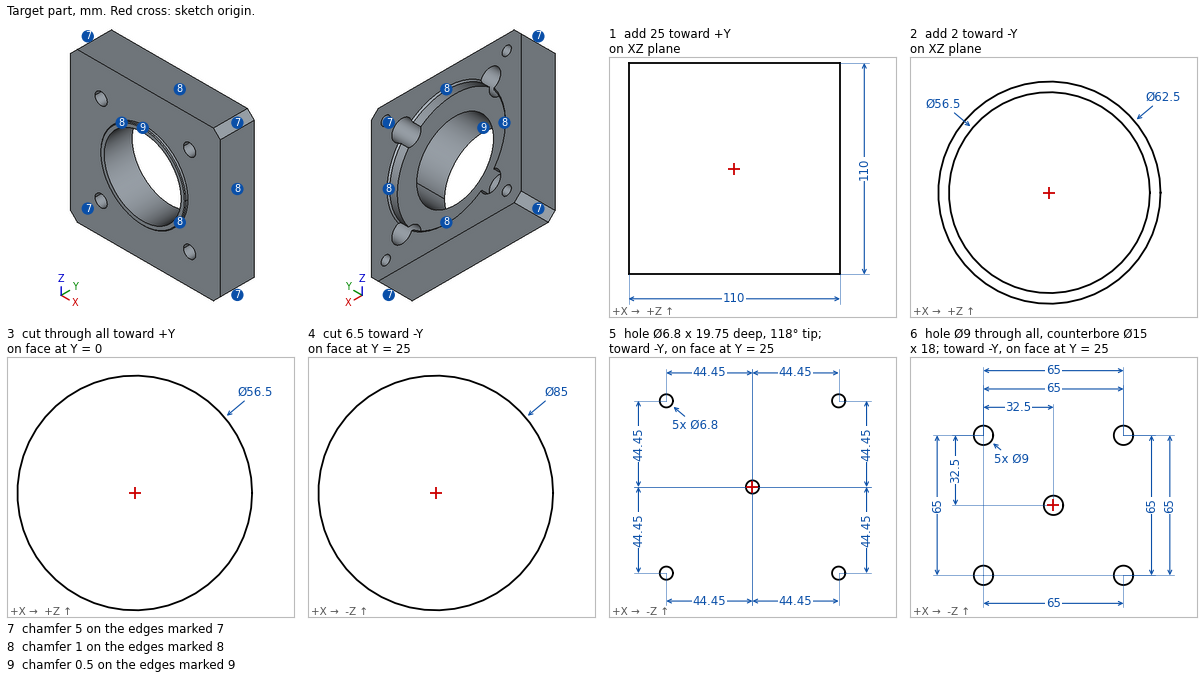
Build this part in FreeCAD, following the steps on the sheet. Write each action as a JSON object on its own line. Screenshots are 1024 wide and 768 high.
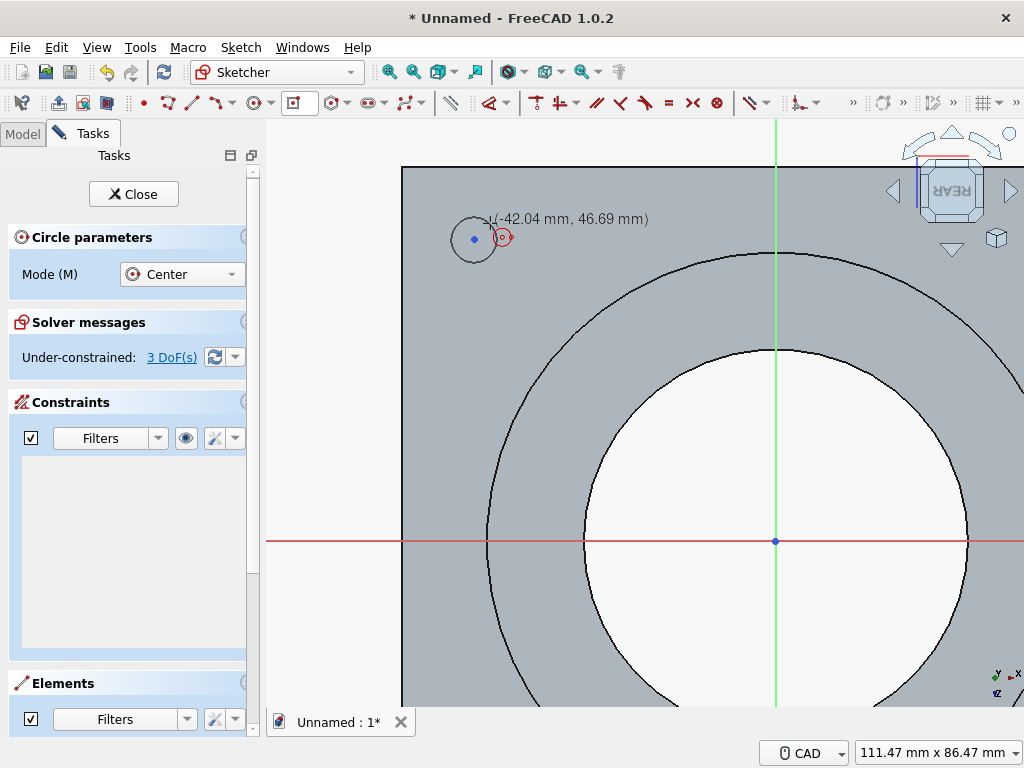
{"action": "left_click", "coordinate": [776, 541]}
{"action": "left_click", "coordinate": [792, 525]}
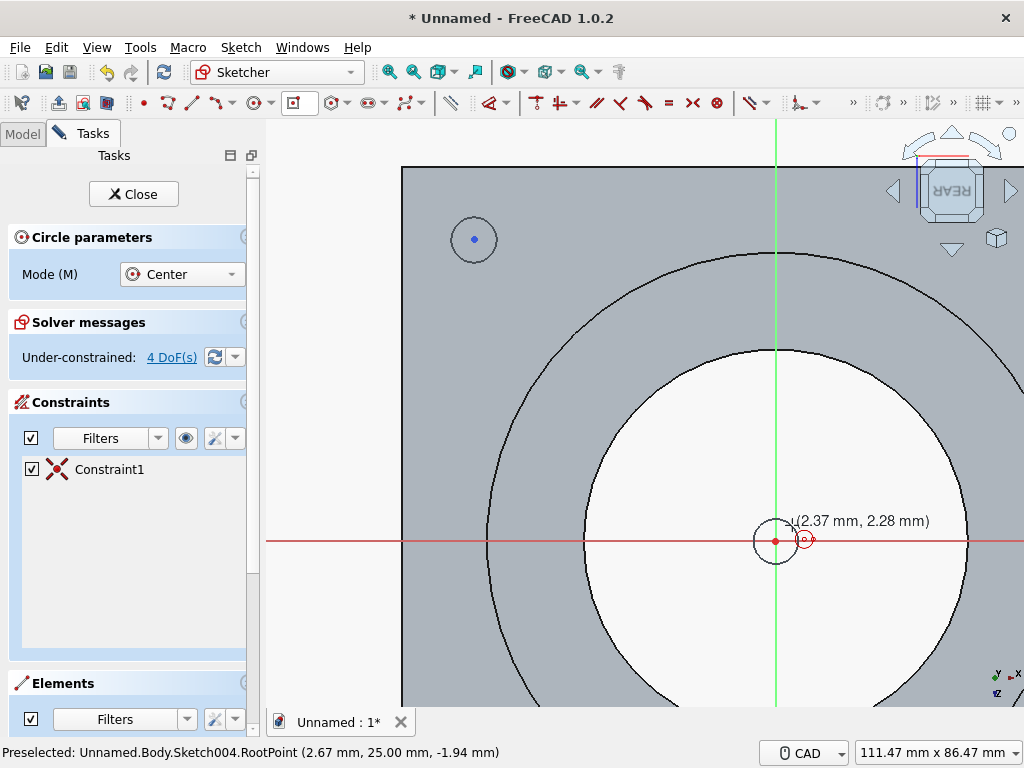
{"action": "scroll", "coordinate": [334, 257], "scroll_direction": "down", "scroll_amount": 3}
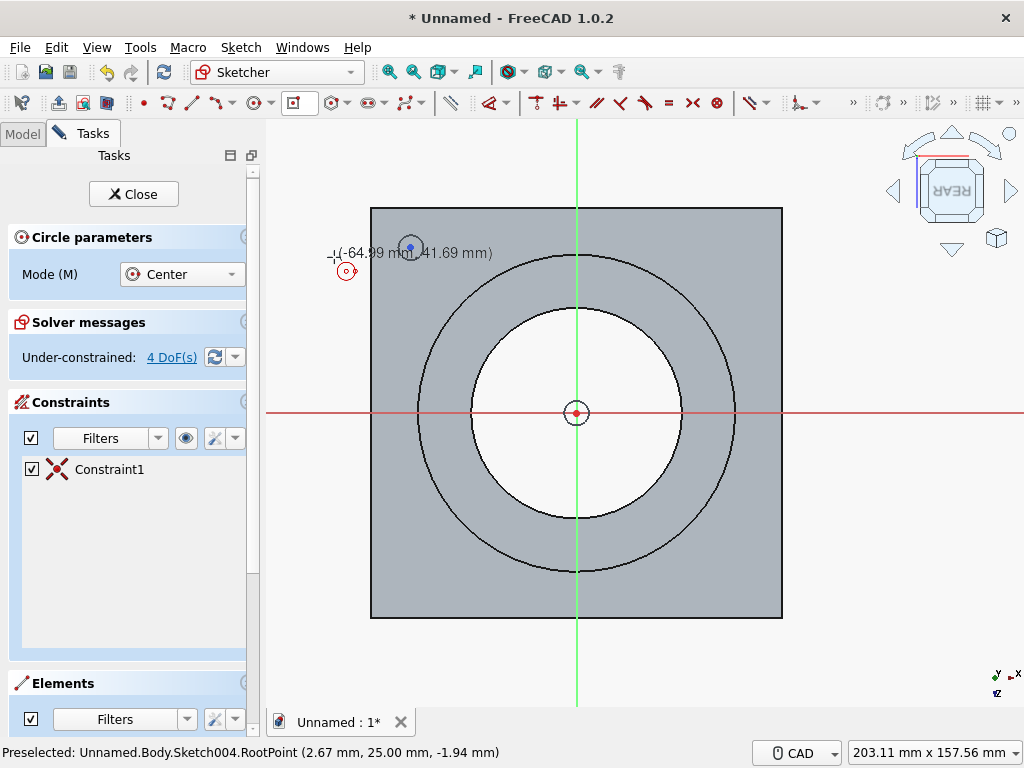
{"action": "scroll", "coordinate": [742, 247], "scroll_direction": "up", "scroll_amount": 3}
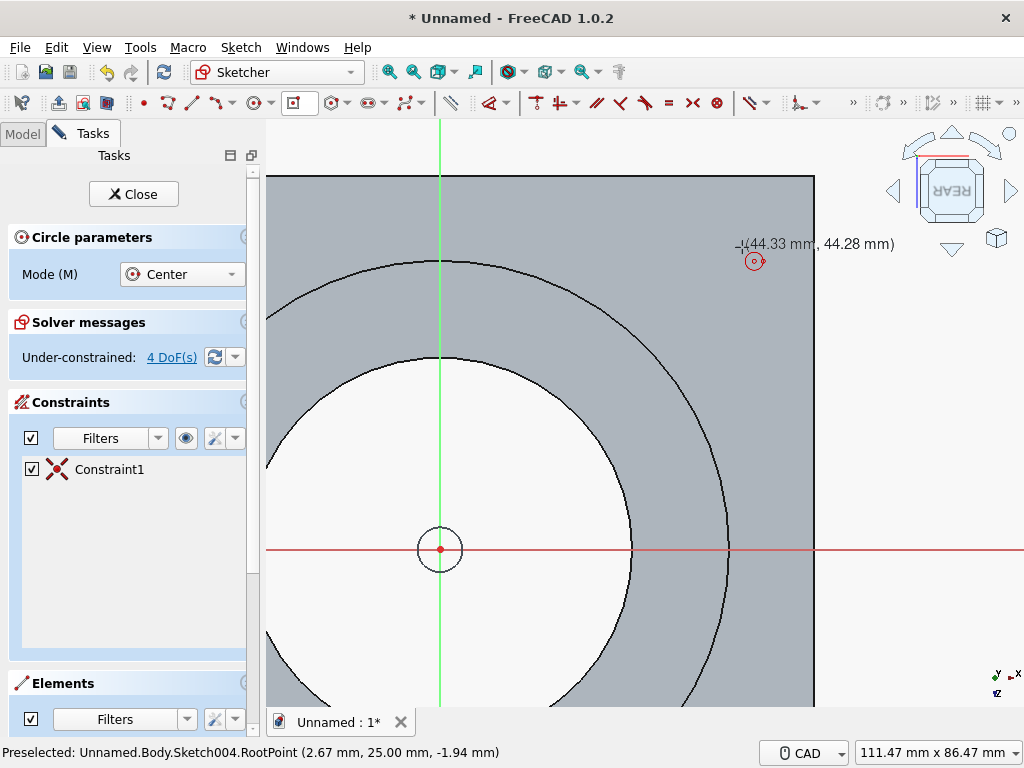
{"action": "left_click", "coordinate": [742, 247]}
{"action": "left_click", "coordinate": [759, 231]}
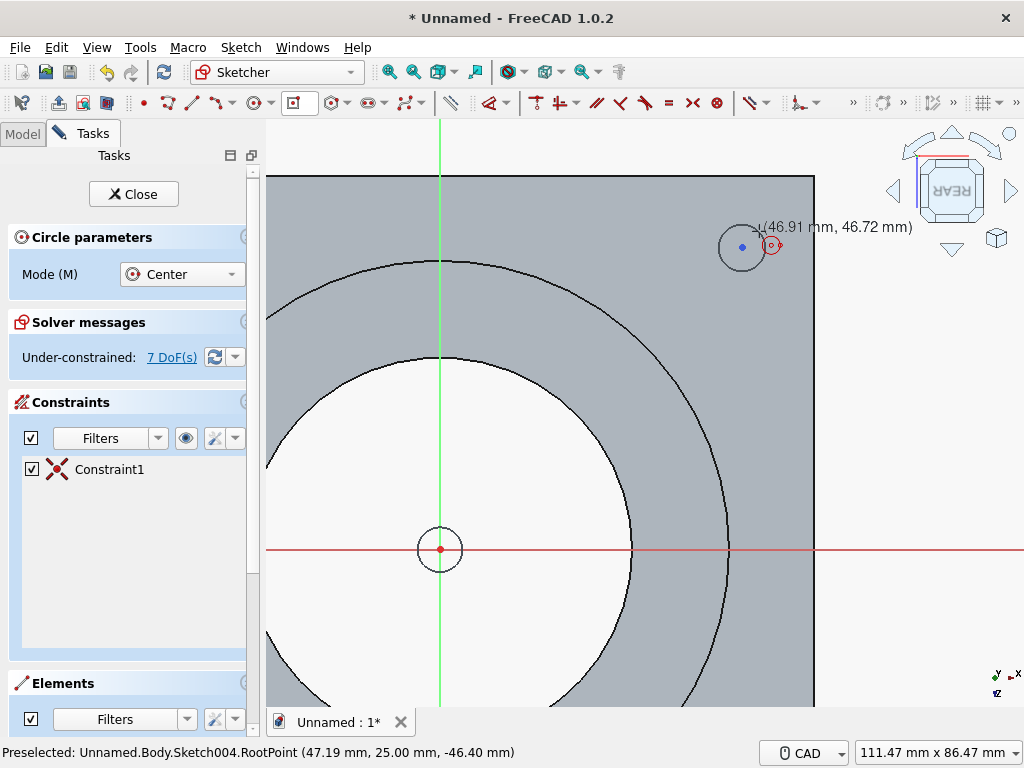
{"action": "scroll", "coordinate": [742, 247], "scroll_direction": "down", "scroll_amount": 3}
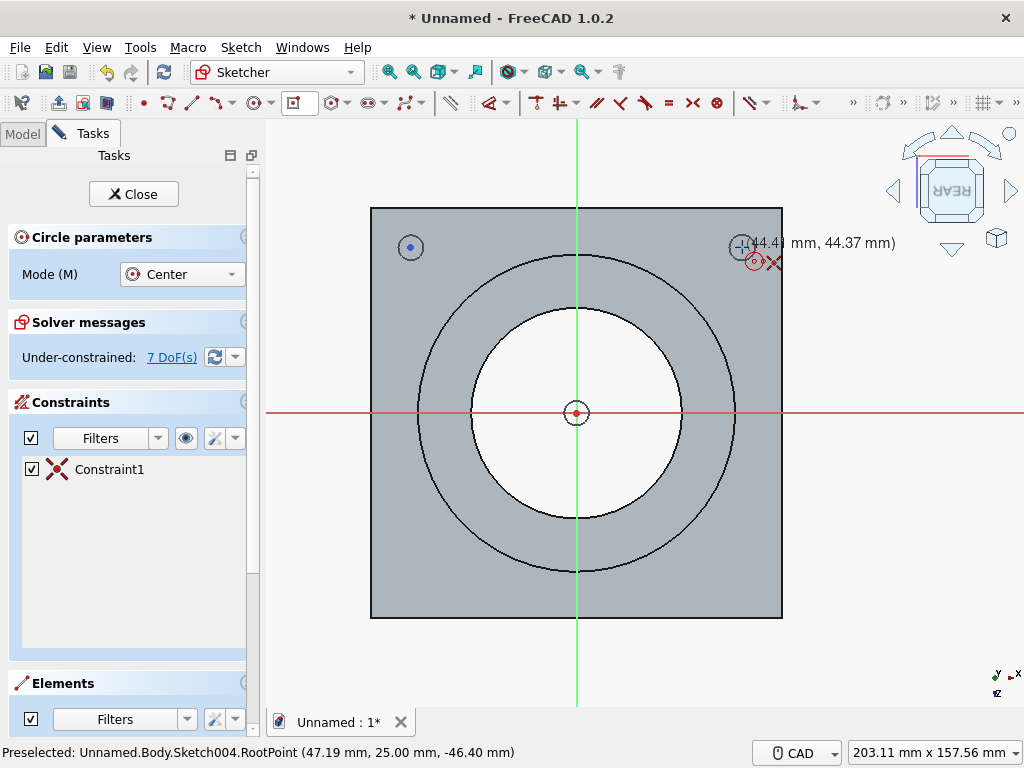
{"action": "scroll", "coordinate": [411, 579], "scroll_direction": "up", "scroll_amount": 3}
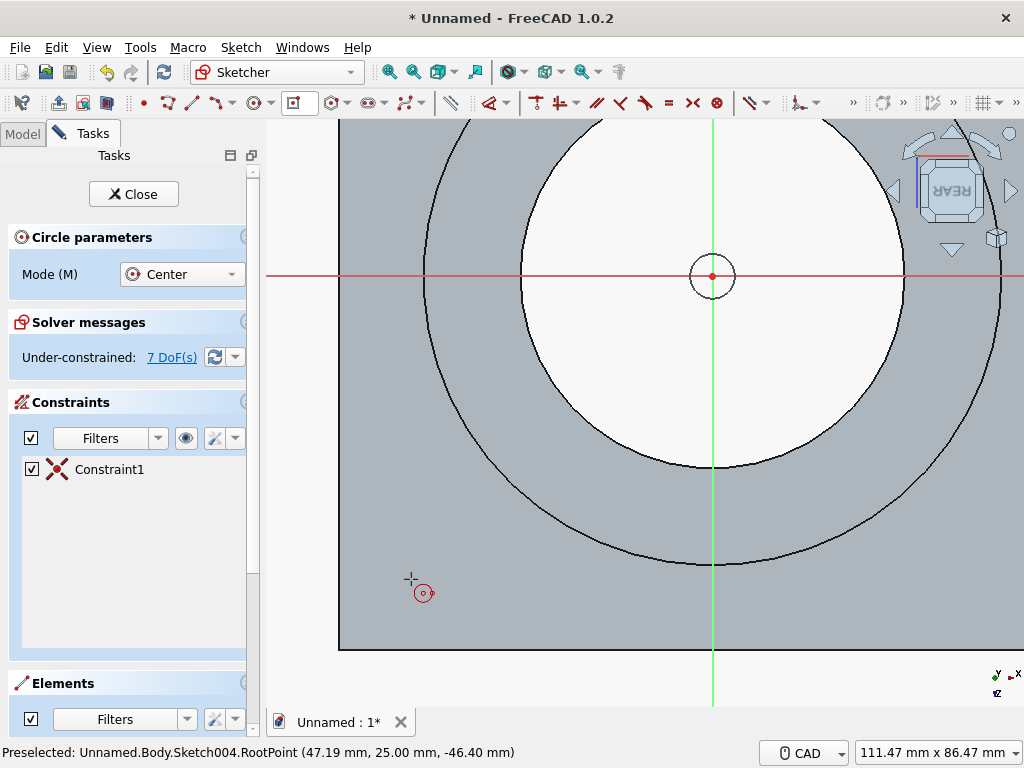
{"action": "left_click", "coordinate": [410, 579]}
{"action": "left_click", "coordinate": [427, 562]}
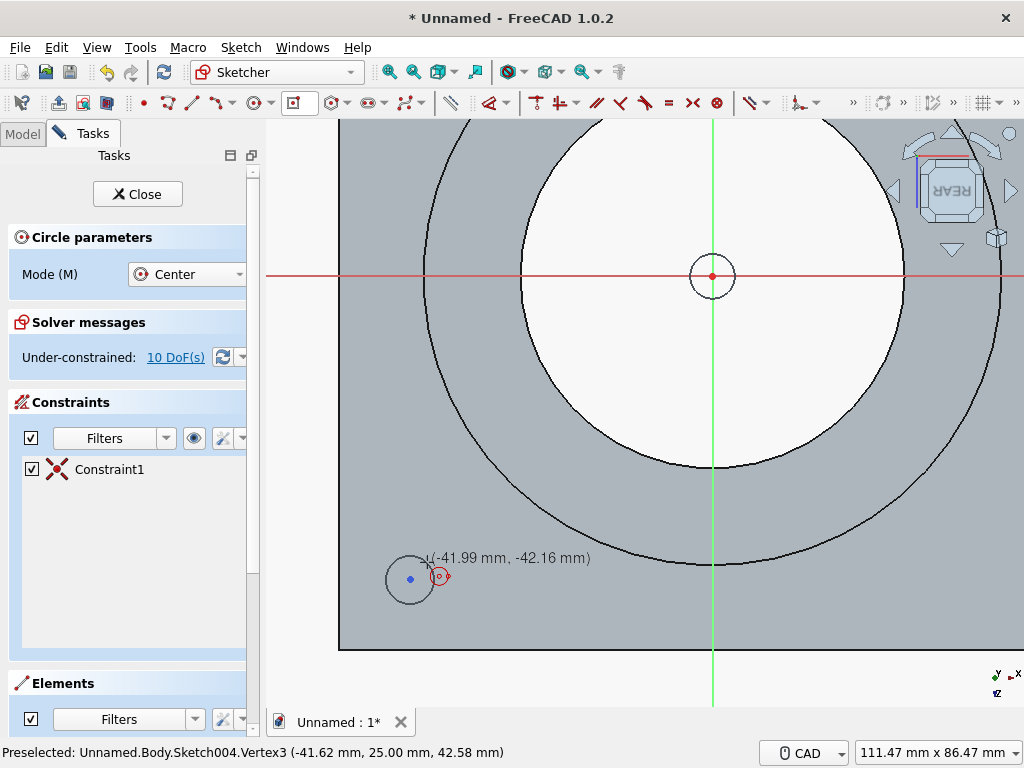
{"action": "scroll", "coordinate": [411, 579], "scroll_direction": "down", "scroll_amount": 3}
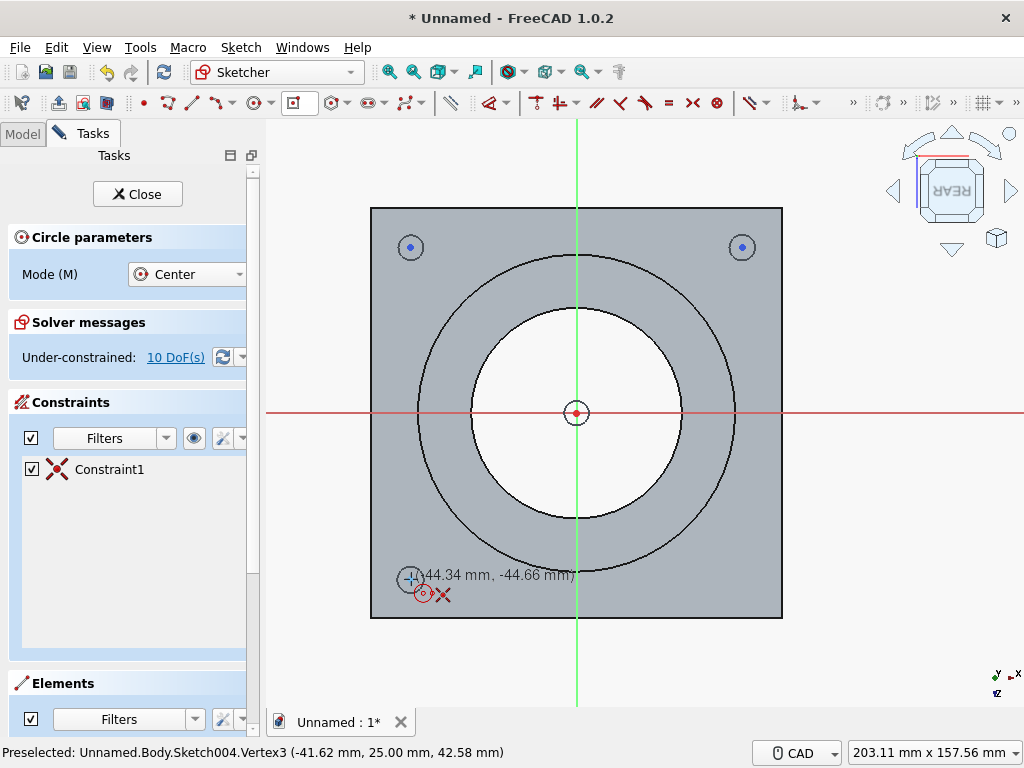
{"action": "scroll", "coordinate": [742, 579], "scroll_direction": "up", "scroll_amount": 3}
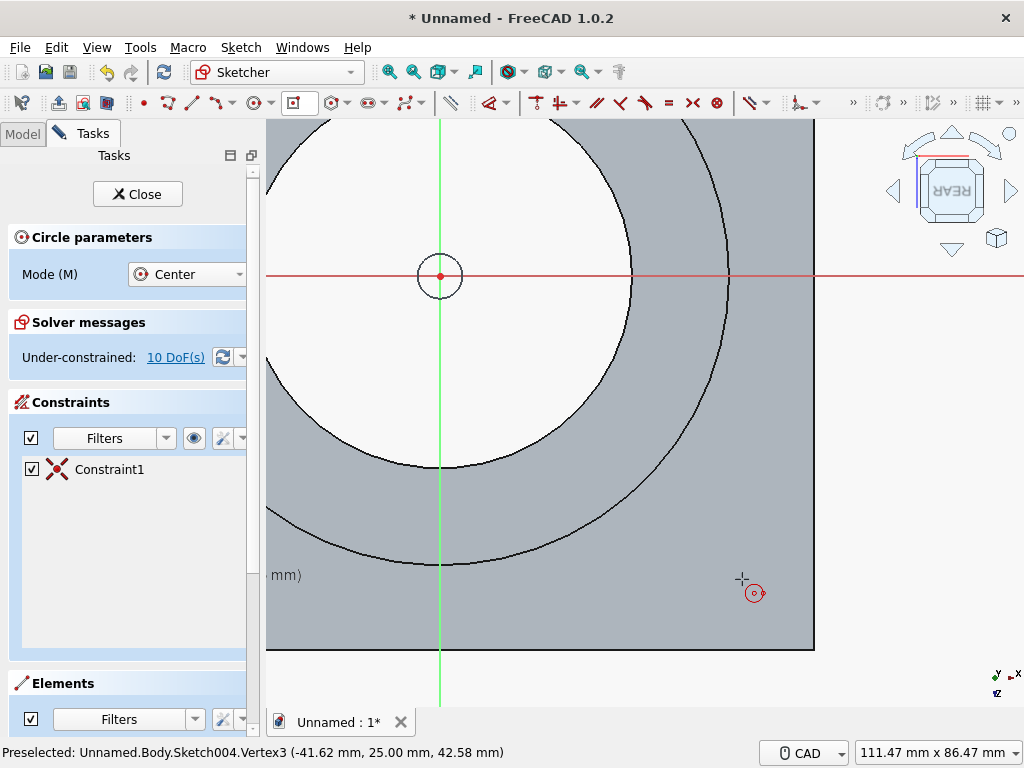
{"action": "left_click", "coordinate": [742, 579]}
{"action": "left_click", "coordinate": [759, 562]}
{"action": "key", "text": "Escape"}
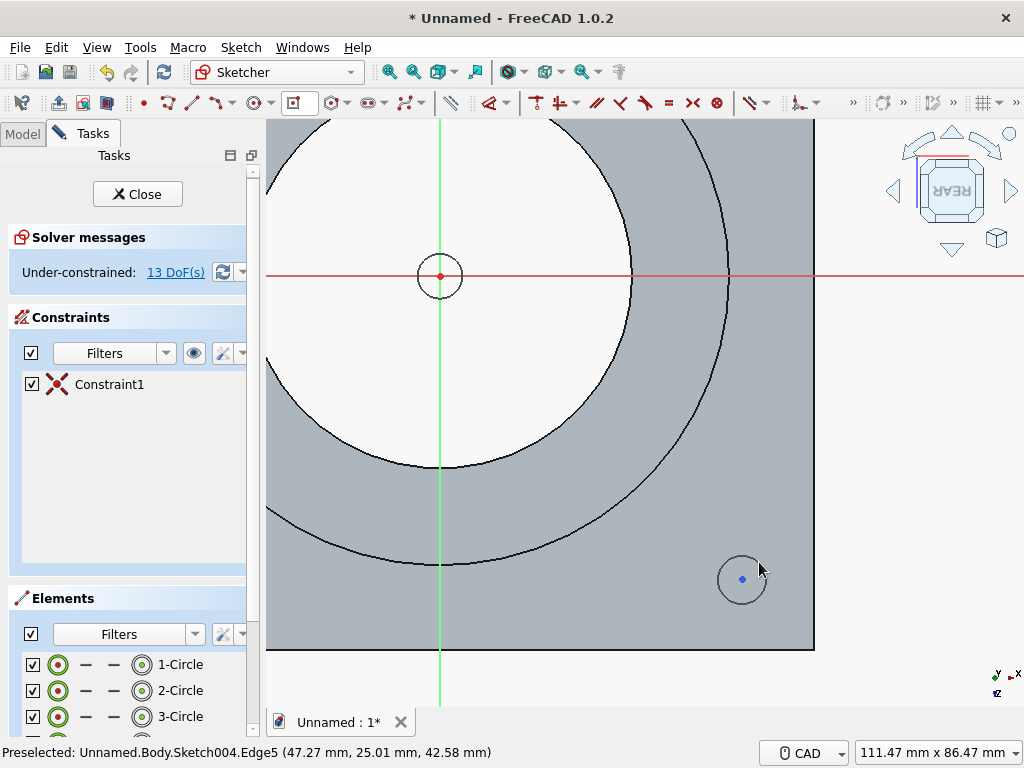
{"action": "scroll", "coordinate": [742, 579], "scroll_direction": "down", "scroll_amount": 3}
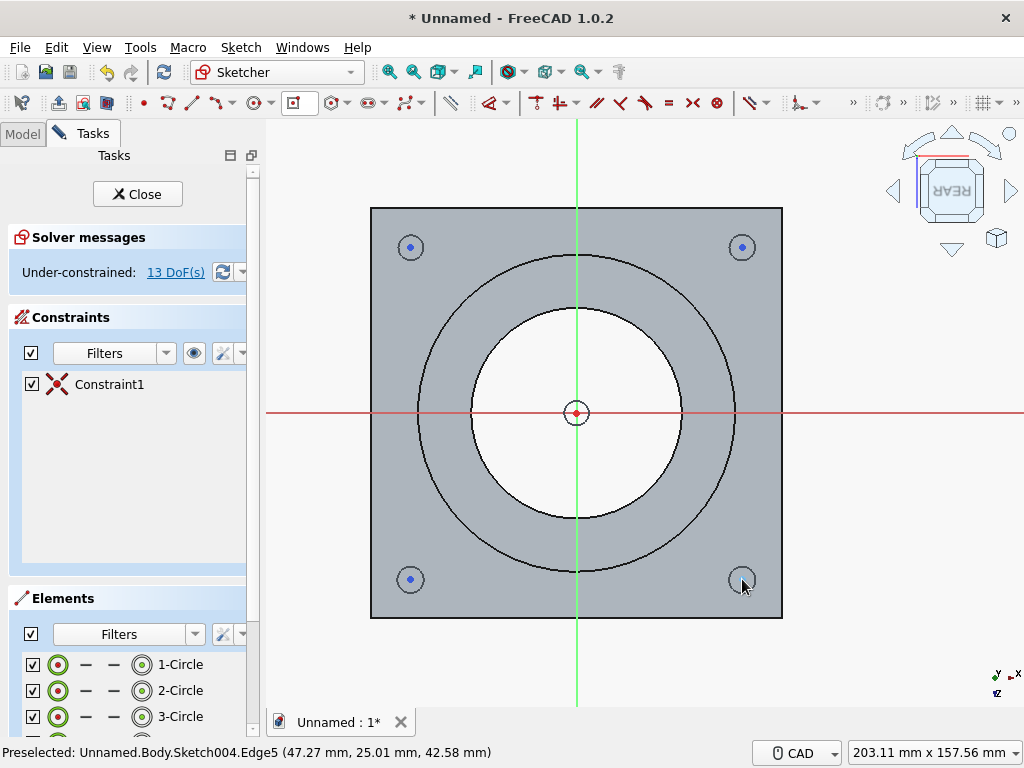
{"action": "left_click", "coordinate": [420, 239]}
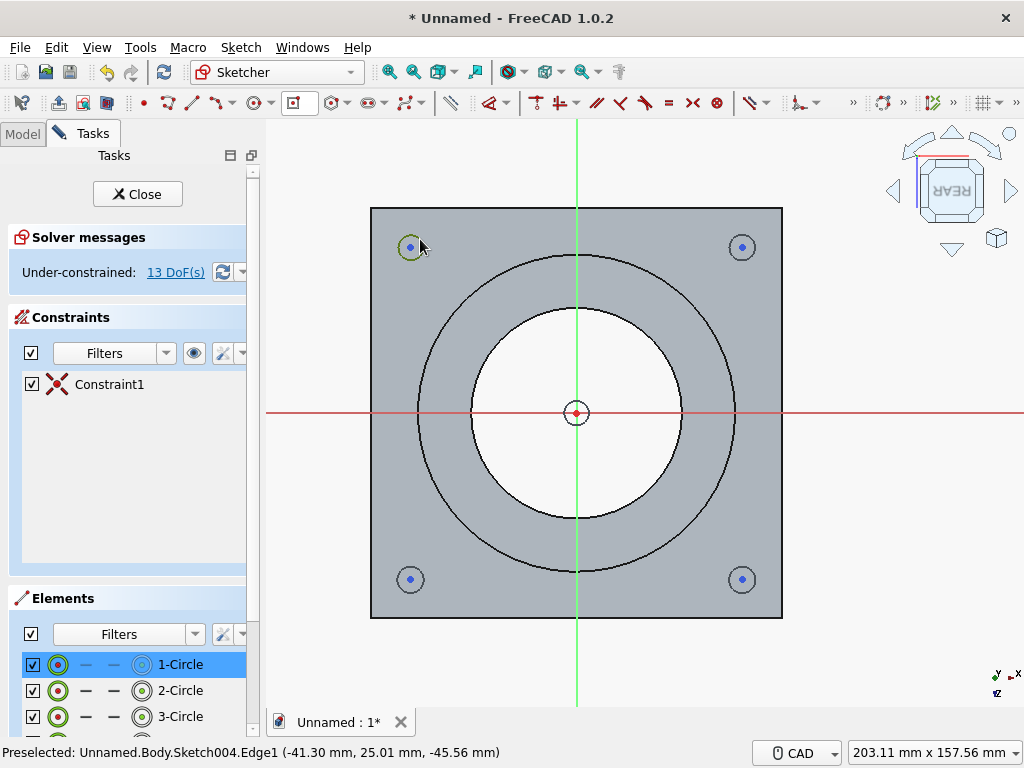
{"action": "left_click", "coordinate": [577, 401]}